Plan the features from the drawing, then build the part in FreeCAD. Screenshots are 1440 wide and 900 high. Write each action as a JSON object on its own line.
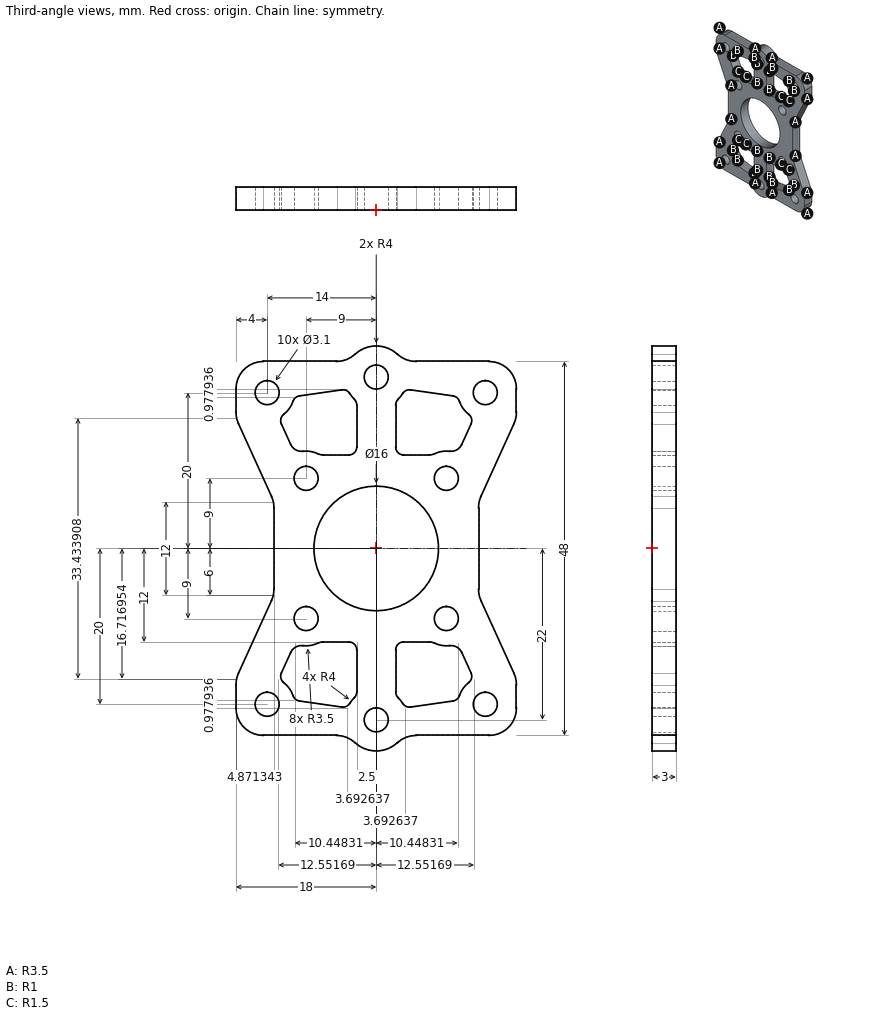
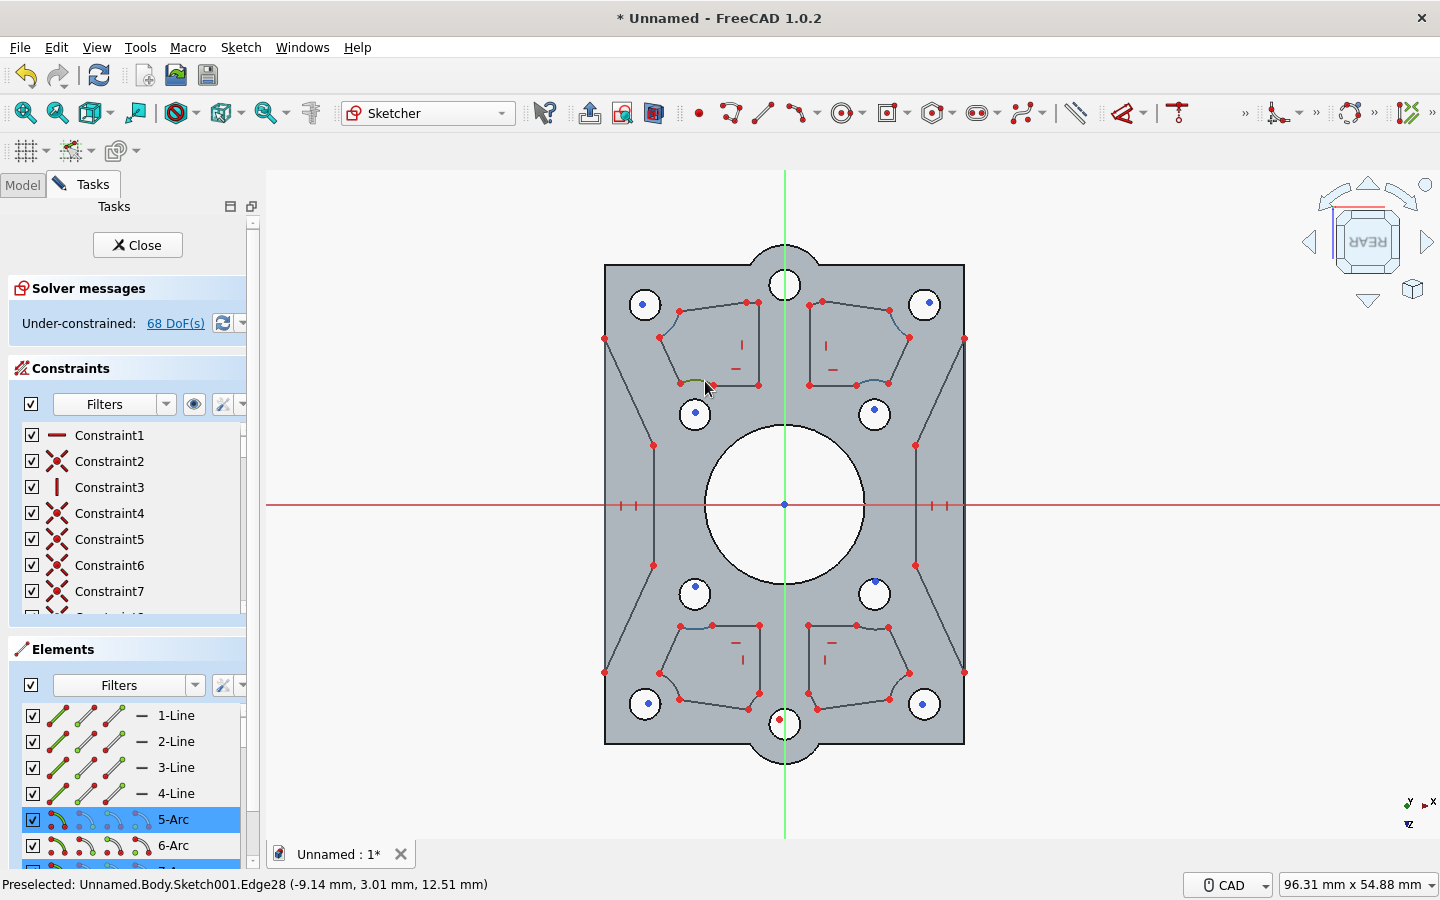
{"action": "scroll", "coordinate": [677, 690], "scroll_direction": "up", "scroll_amount": 2}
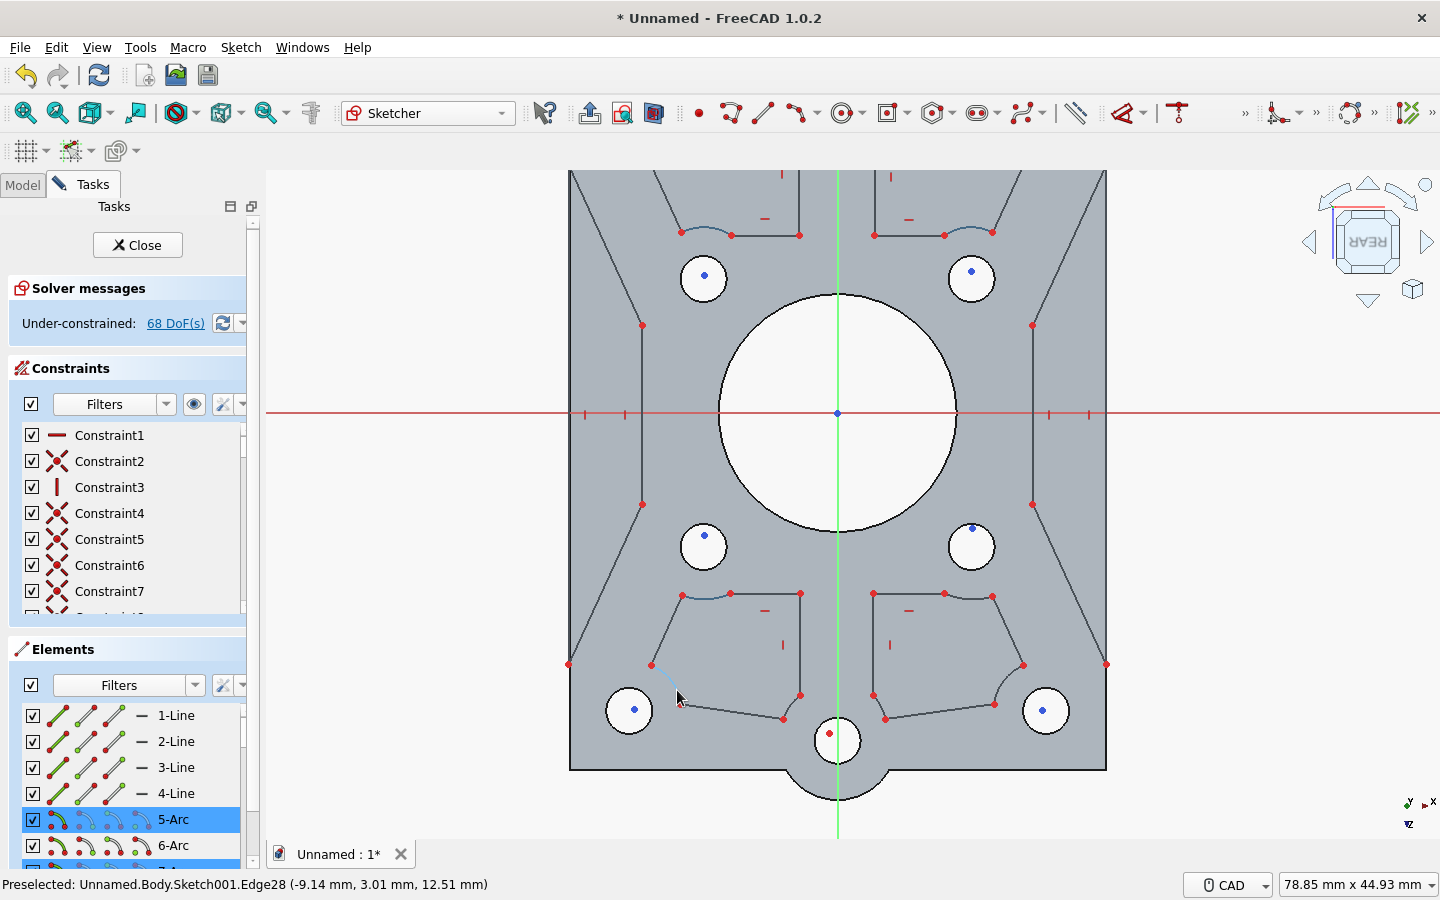
{"action": "left_click", "coordinate": [677, 689]}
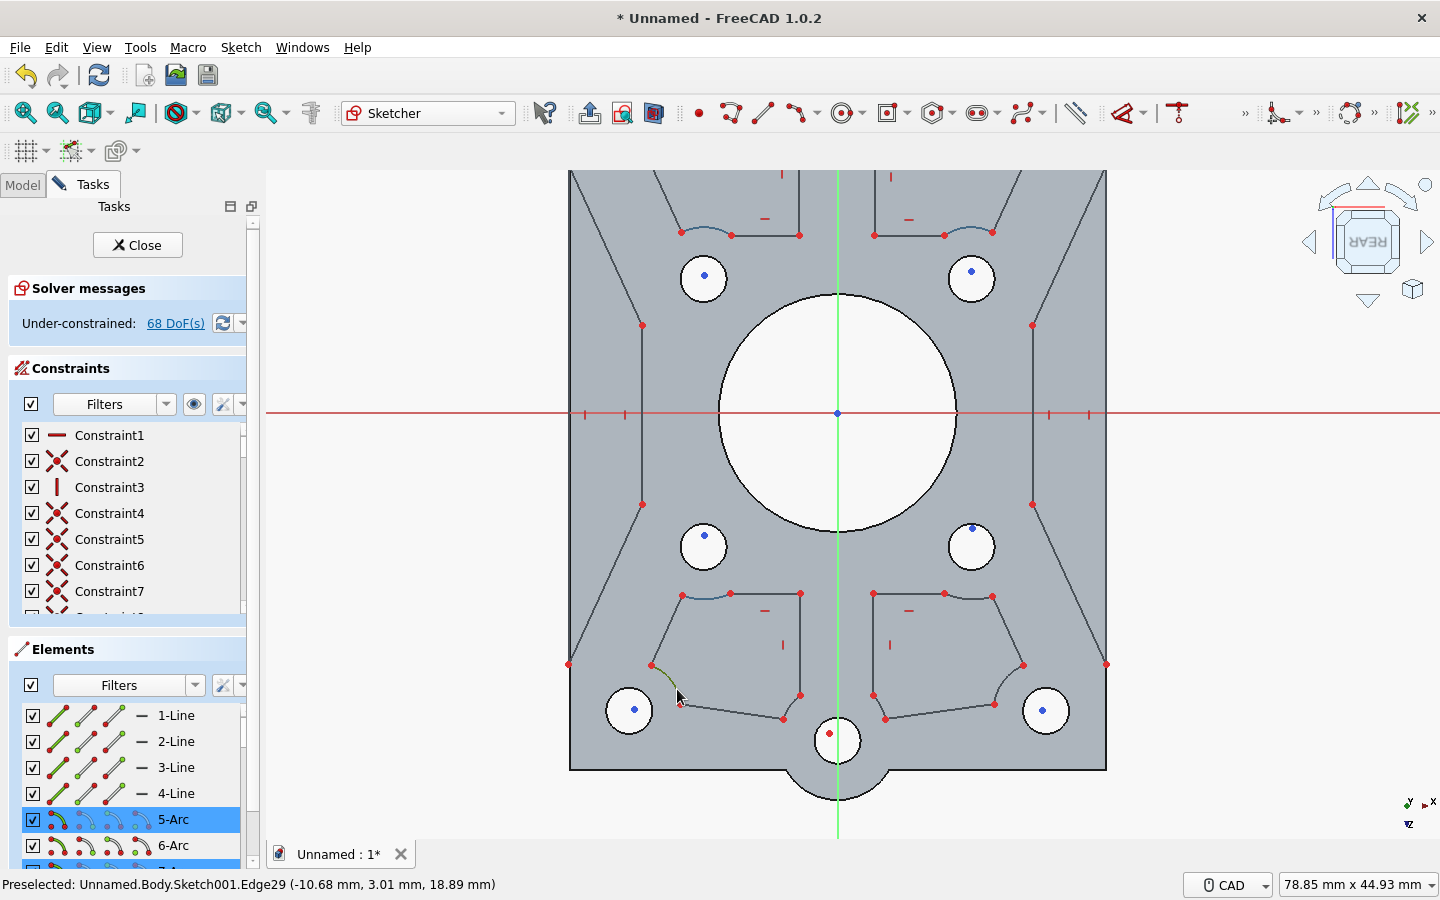
{"action": "left_click", "coordinate": [1011, 673]}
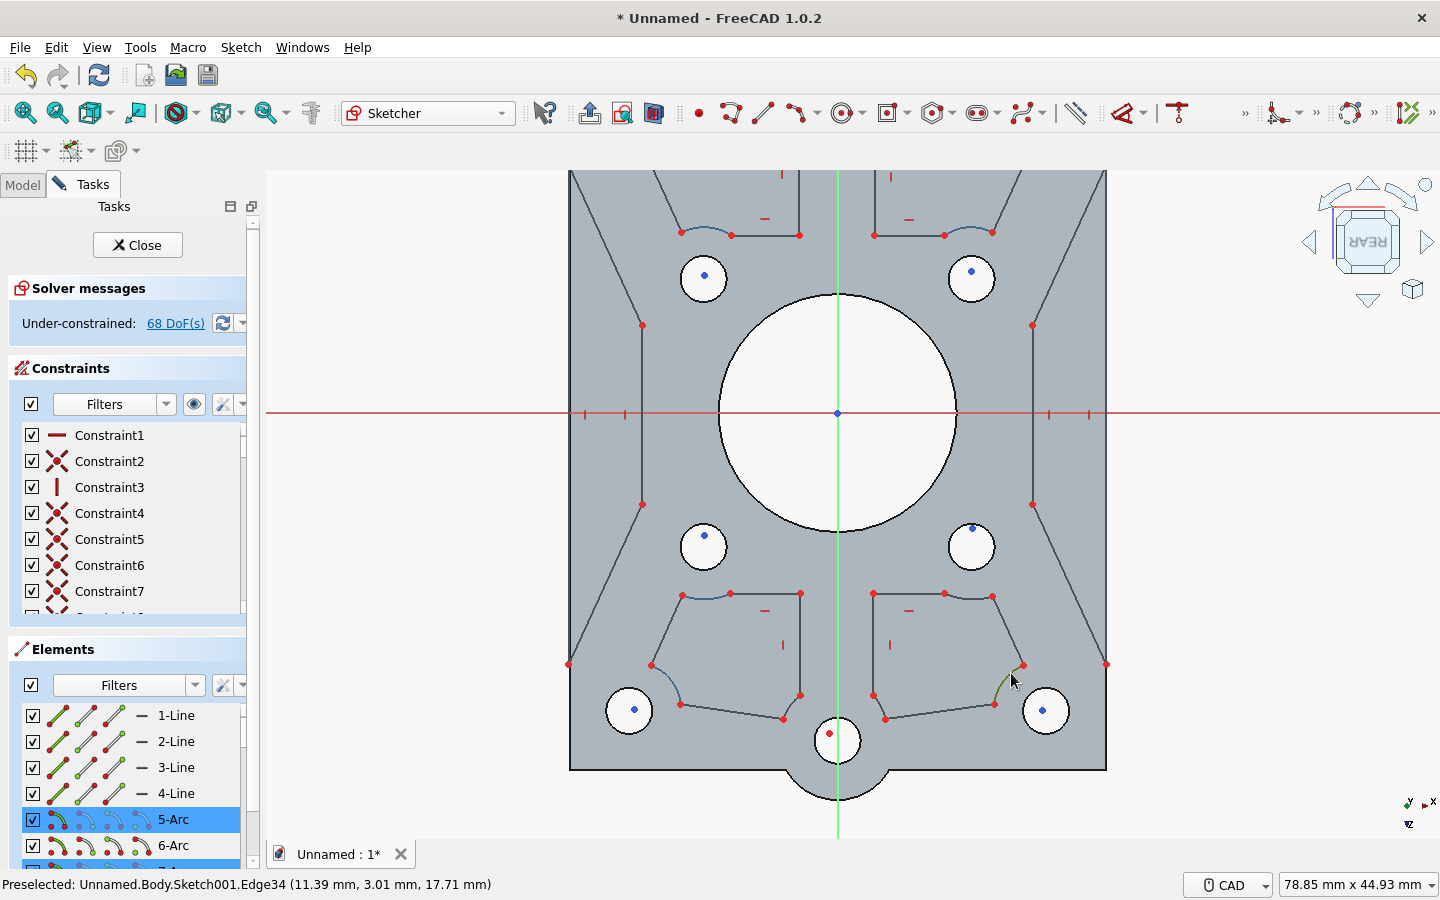
{"action": "left_click", "coordinate": [959, 598]}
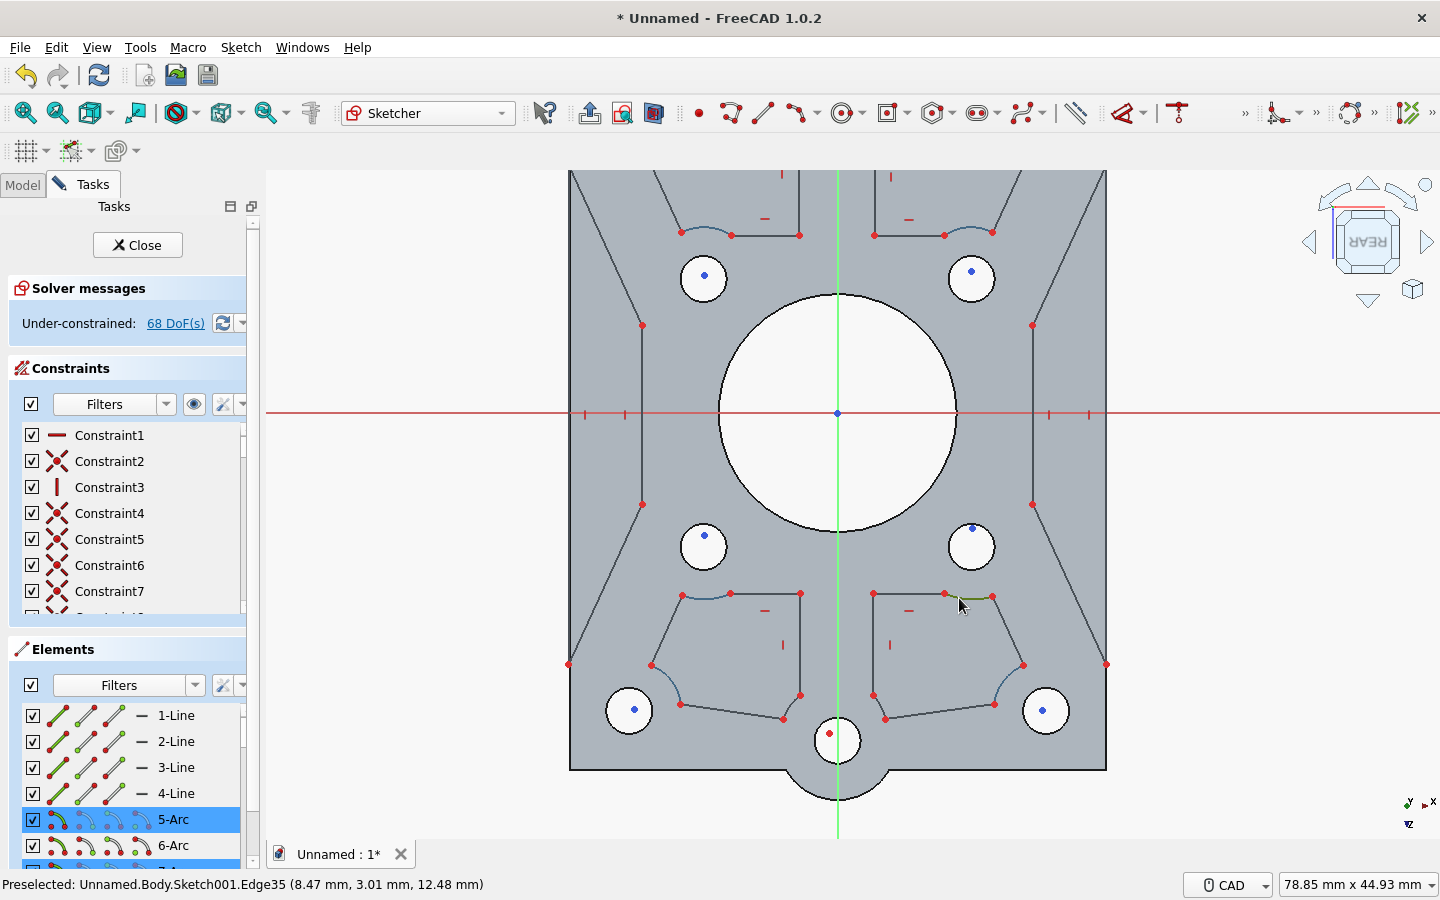
{"action": "key", "text": "e"}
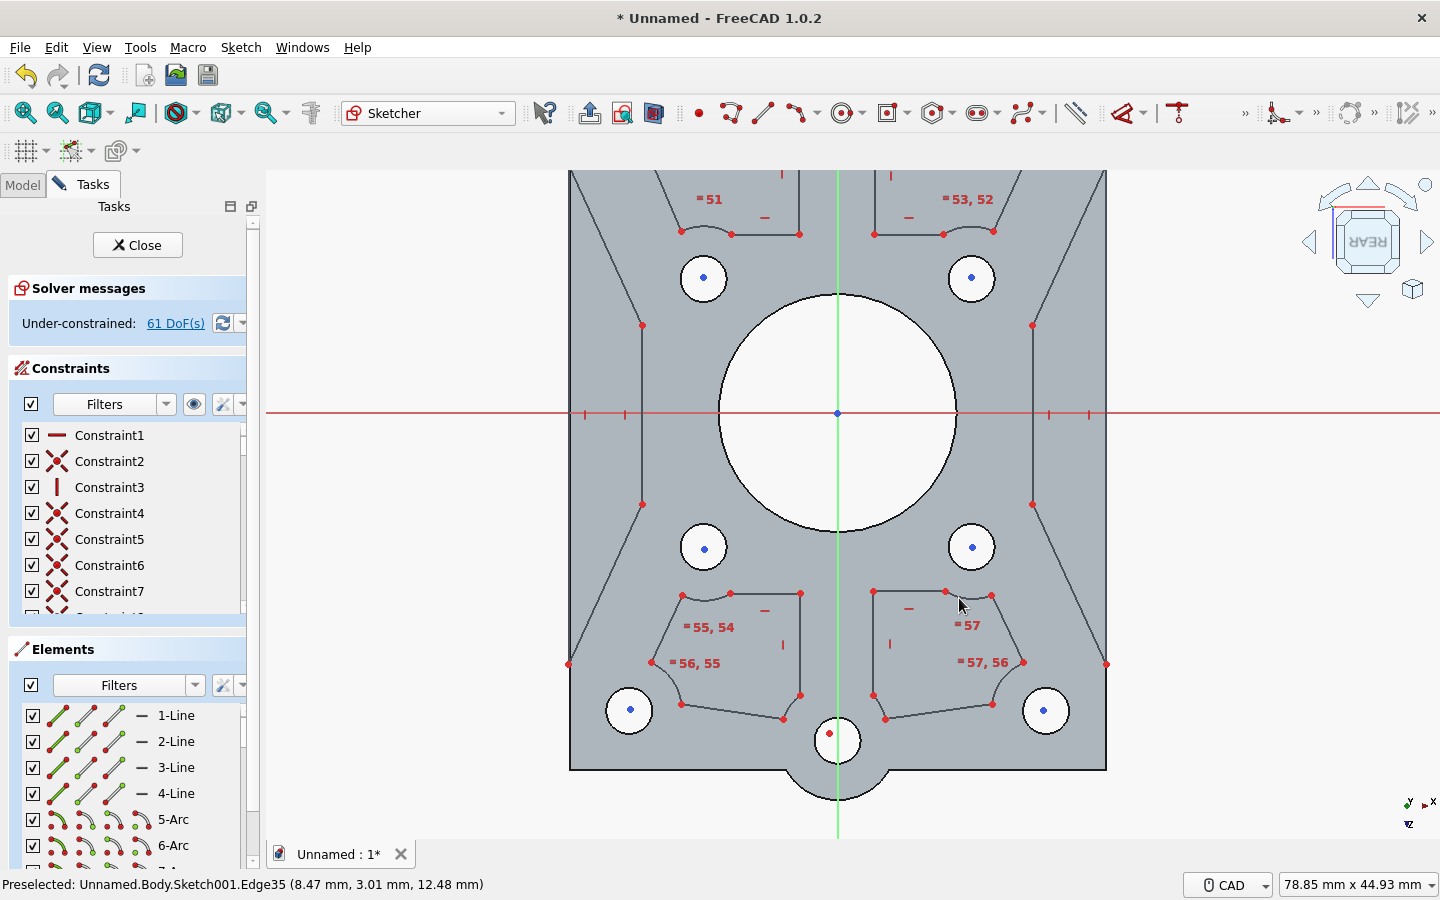
{"action": "scroll", "coordinate": [676, 690], "scroll_direction": "down", "scroll_amount": 2}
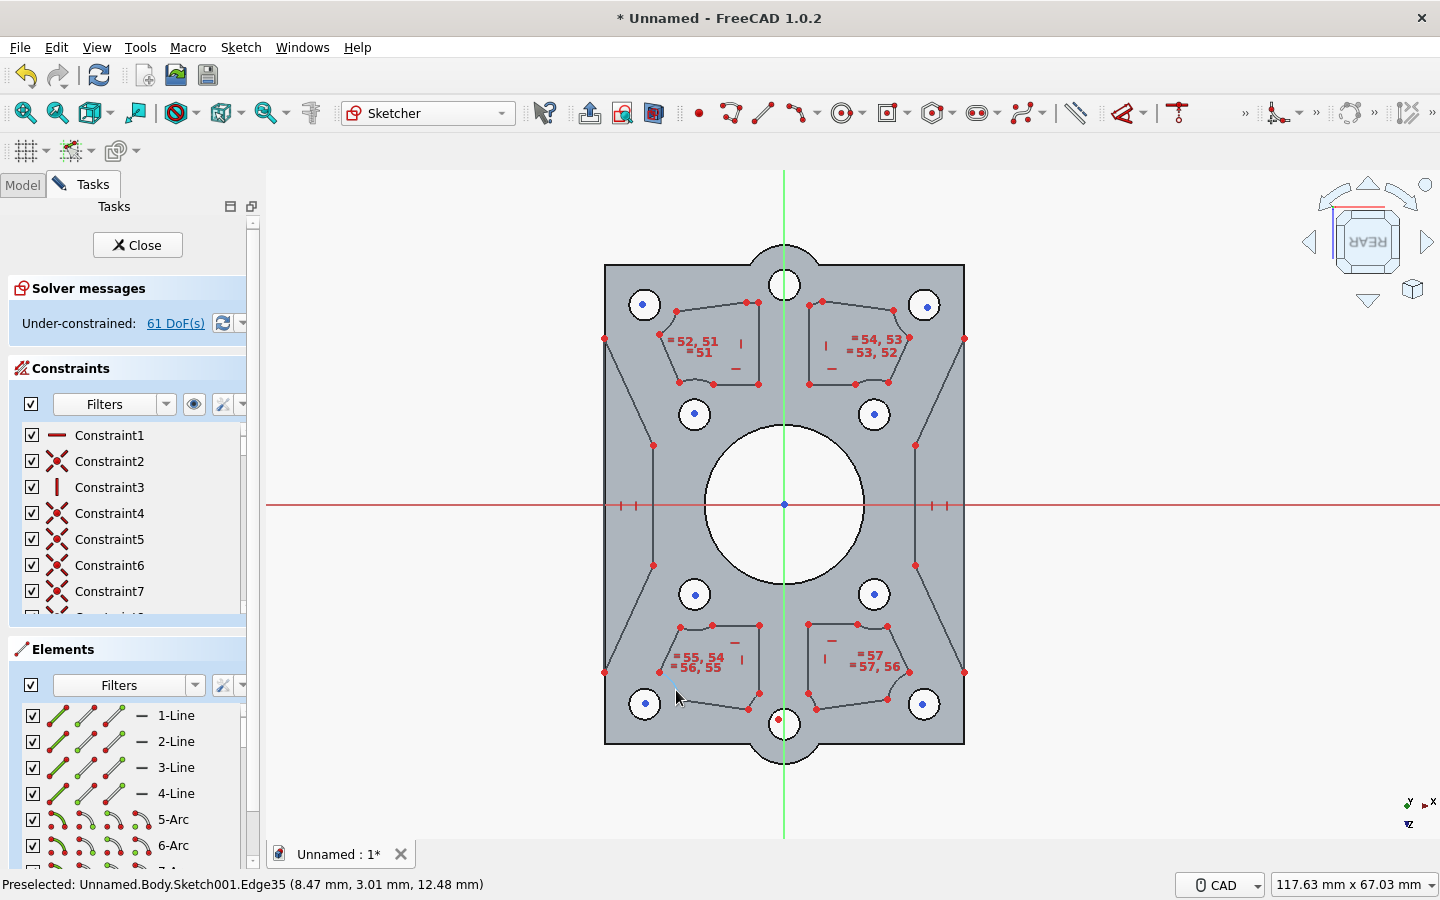
{"action": "scroll", "coordinate": [753, 303], "scroll_direction": "up", "scroll_amount": 5}